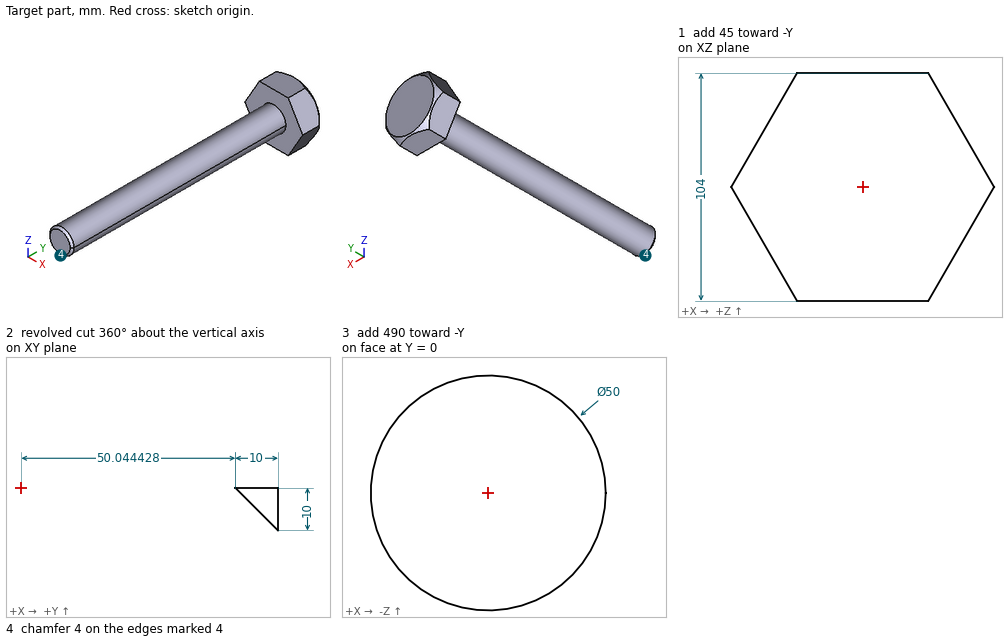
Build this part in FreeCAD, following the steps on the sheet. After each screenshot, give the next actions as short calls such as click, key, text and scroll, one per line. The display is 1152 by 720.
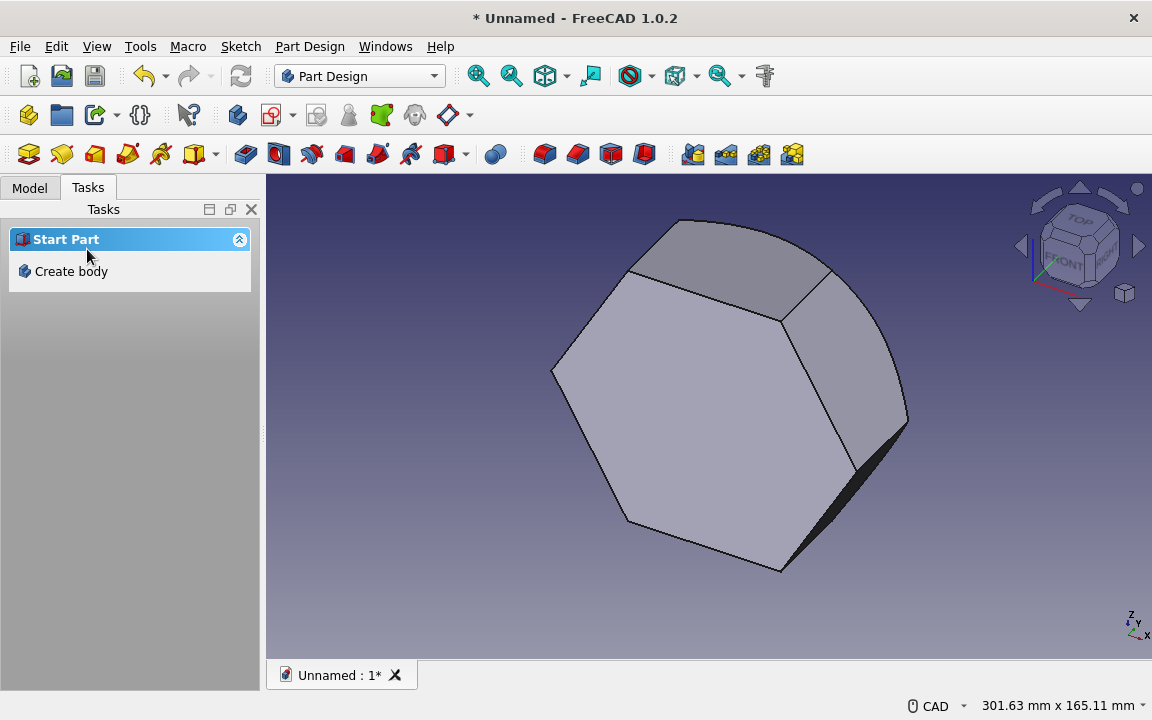
key(4)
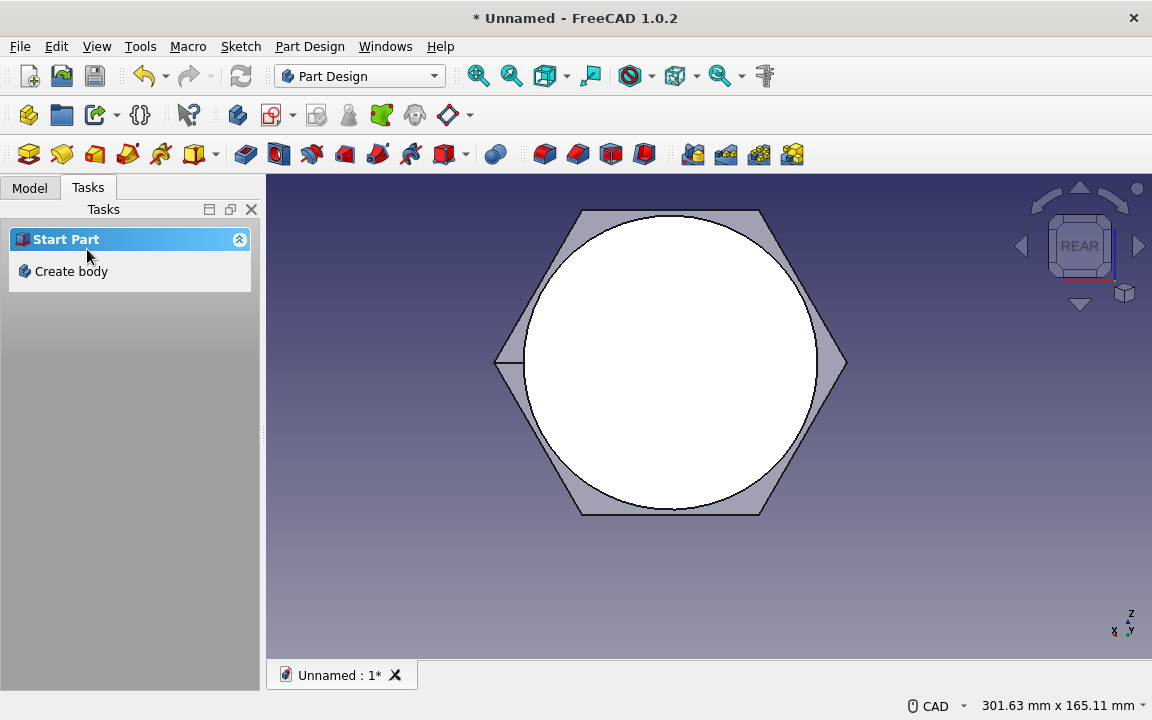
click(671, 362)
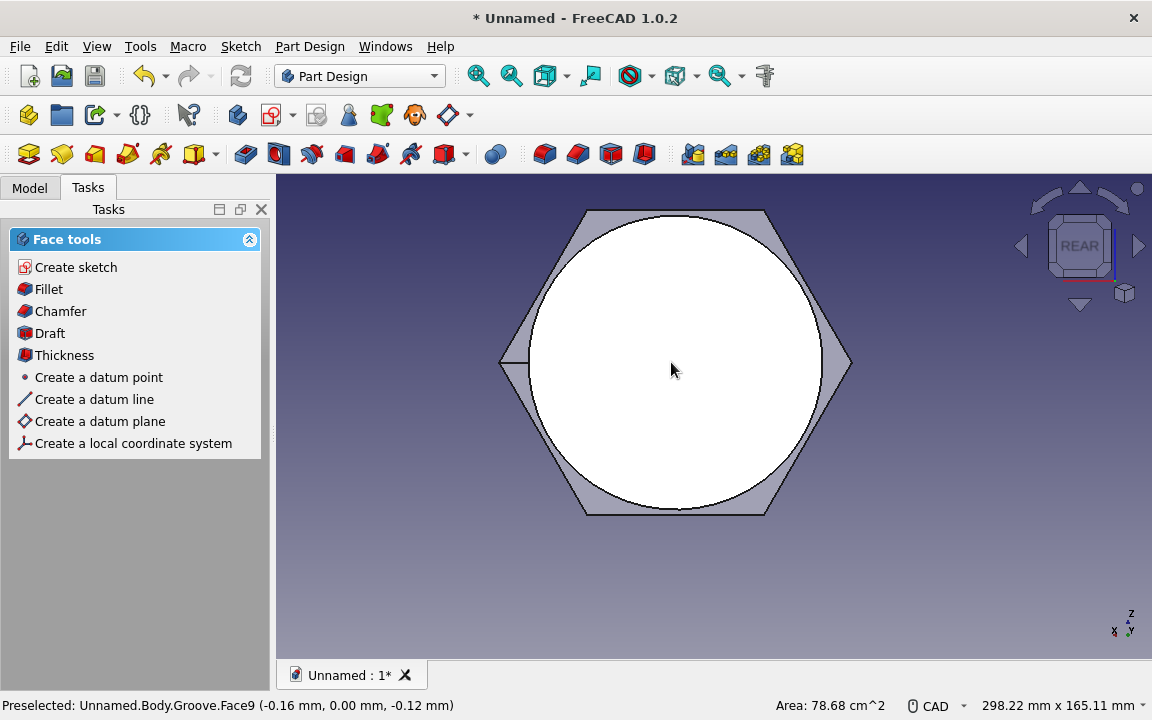
click(270, 116)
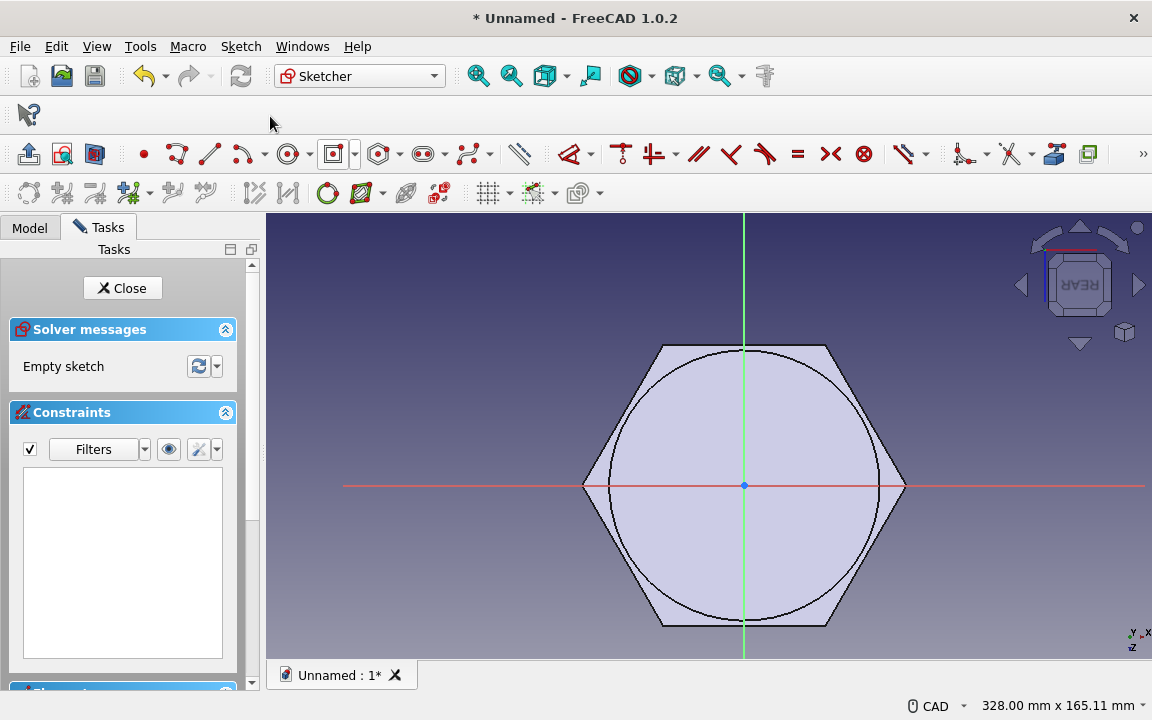
scroll(829, 526, up, 4)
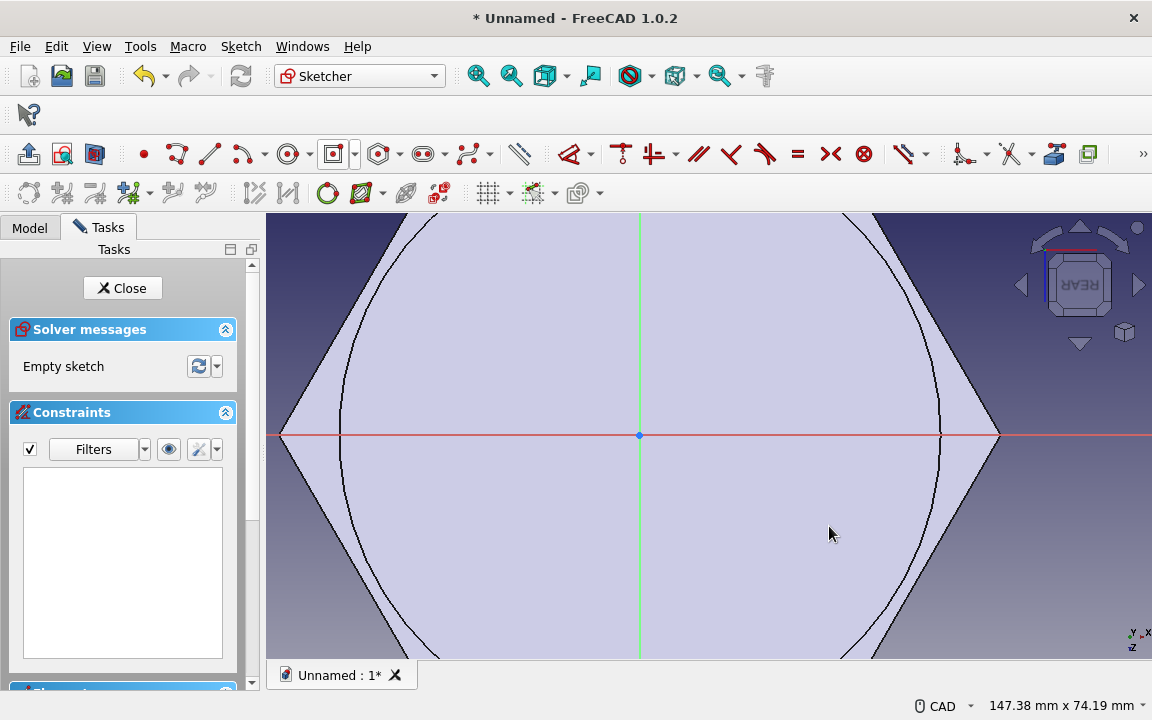
click(288, 154)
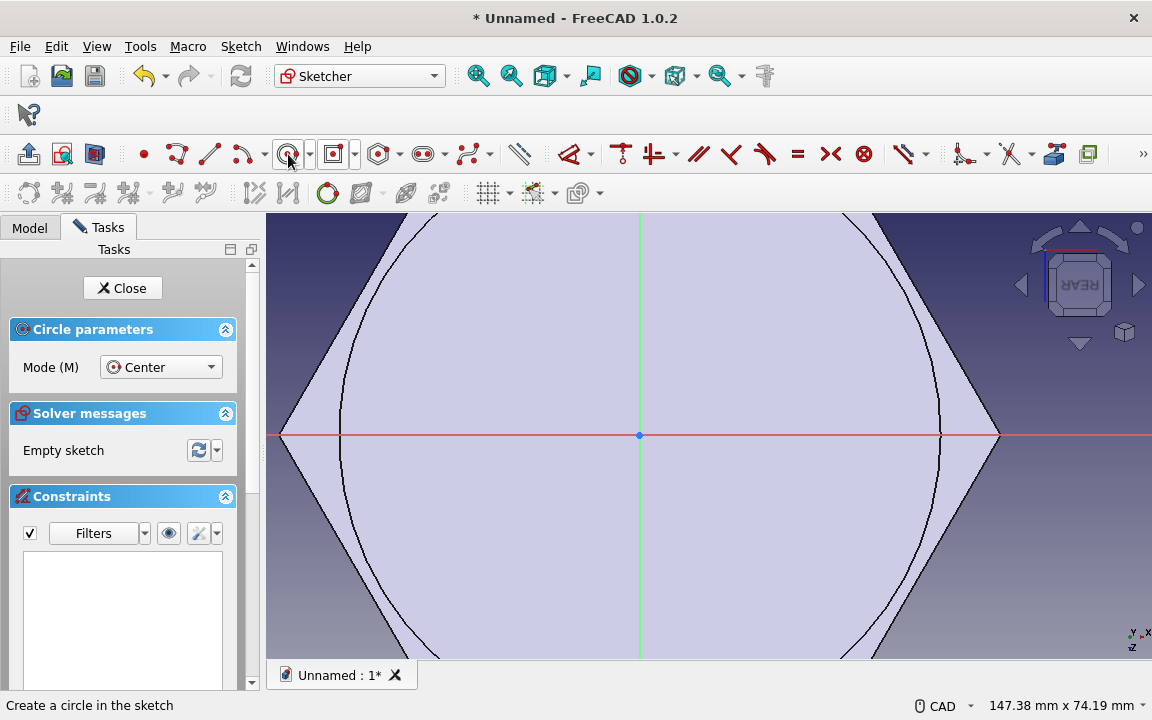
click(640, 435)
move(746, 329)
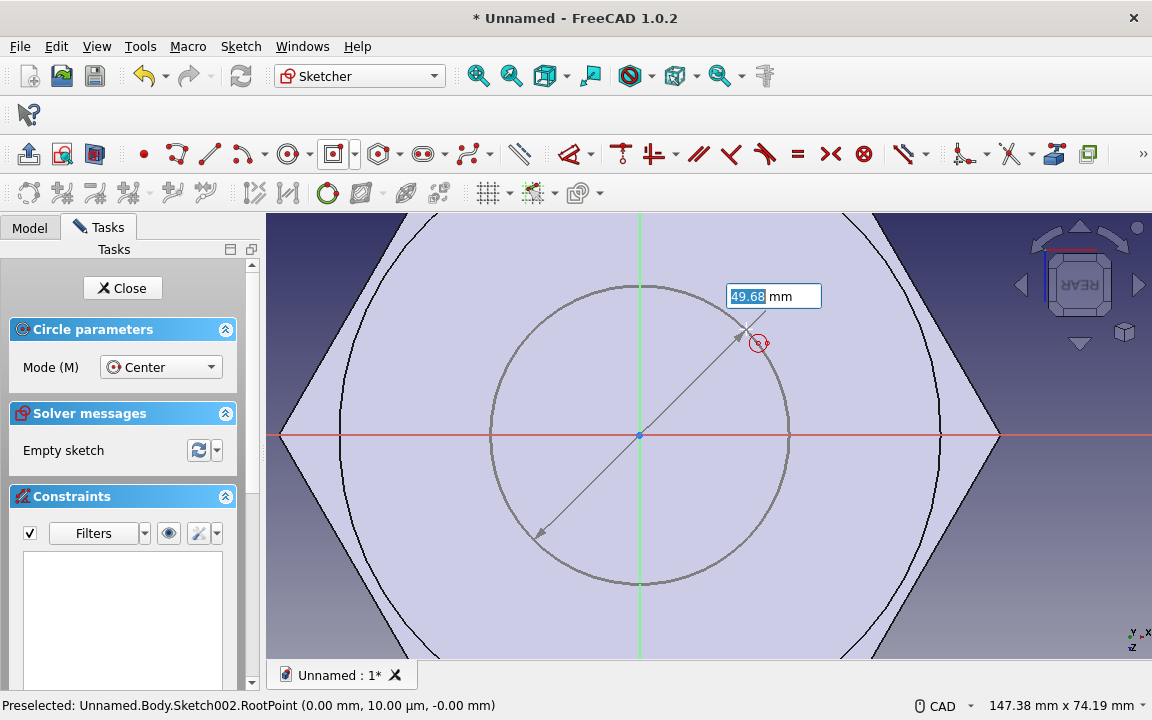
text(50)
key(Return)
key(Escape)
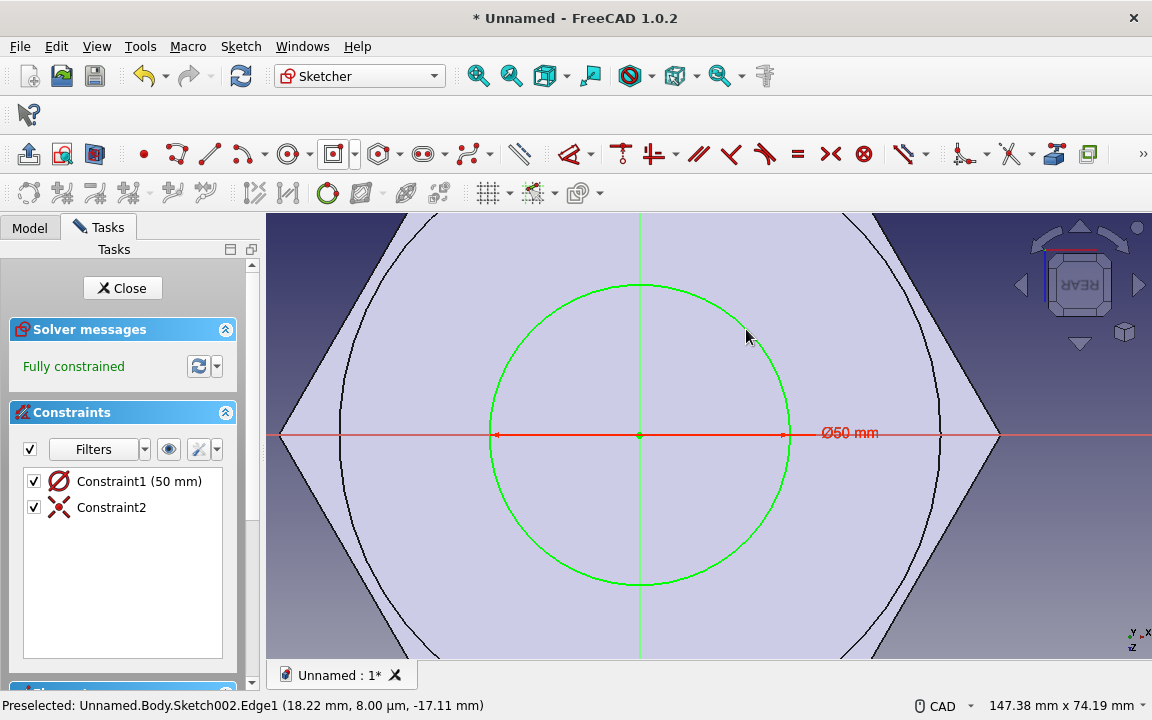
click(123, 288)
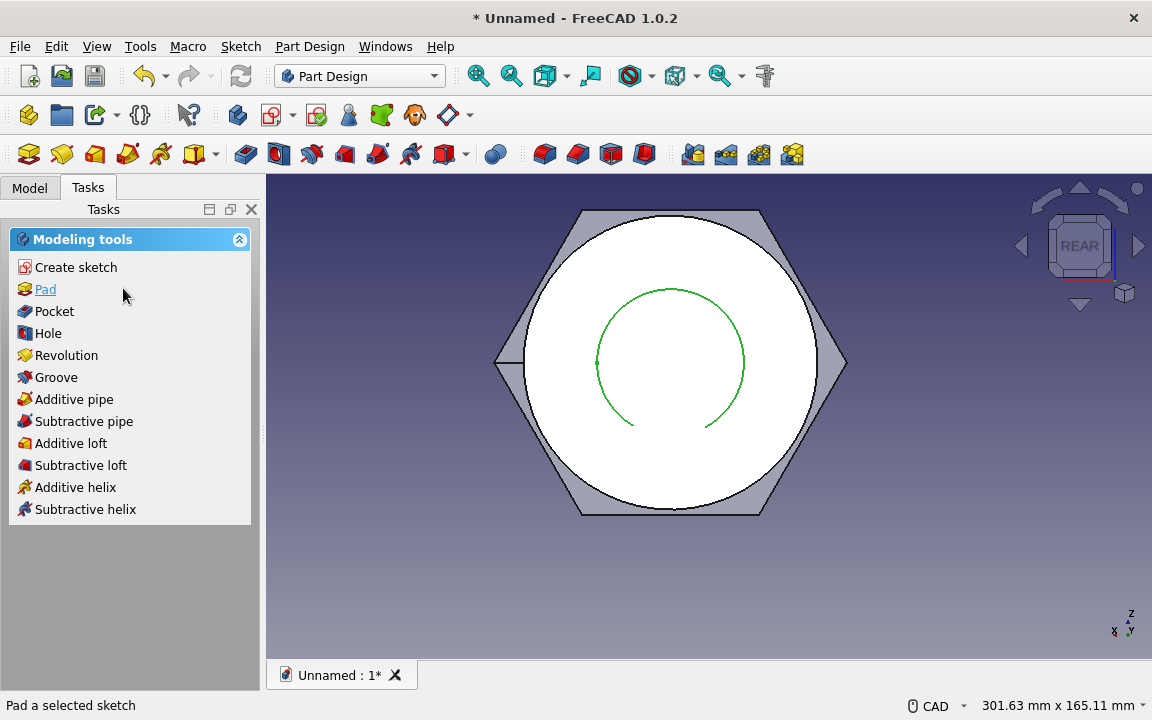
click(29, 154)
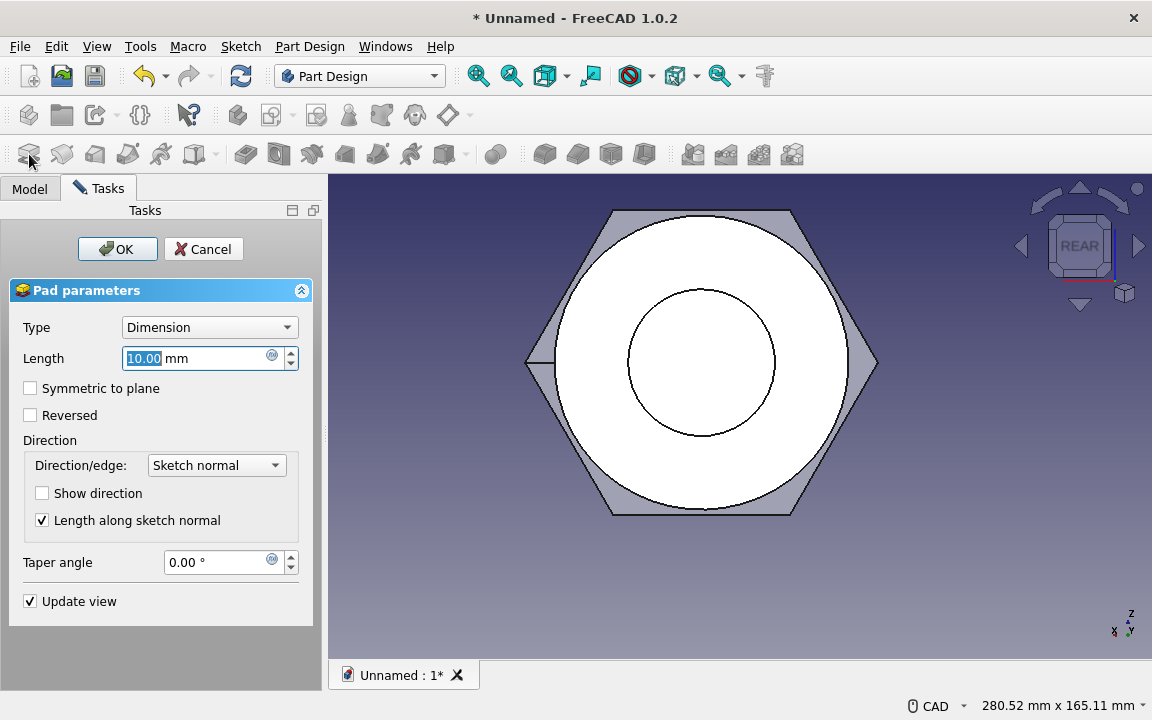
text(490)
key(Tab)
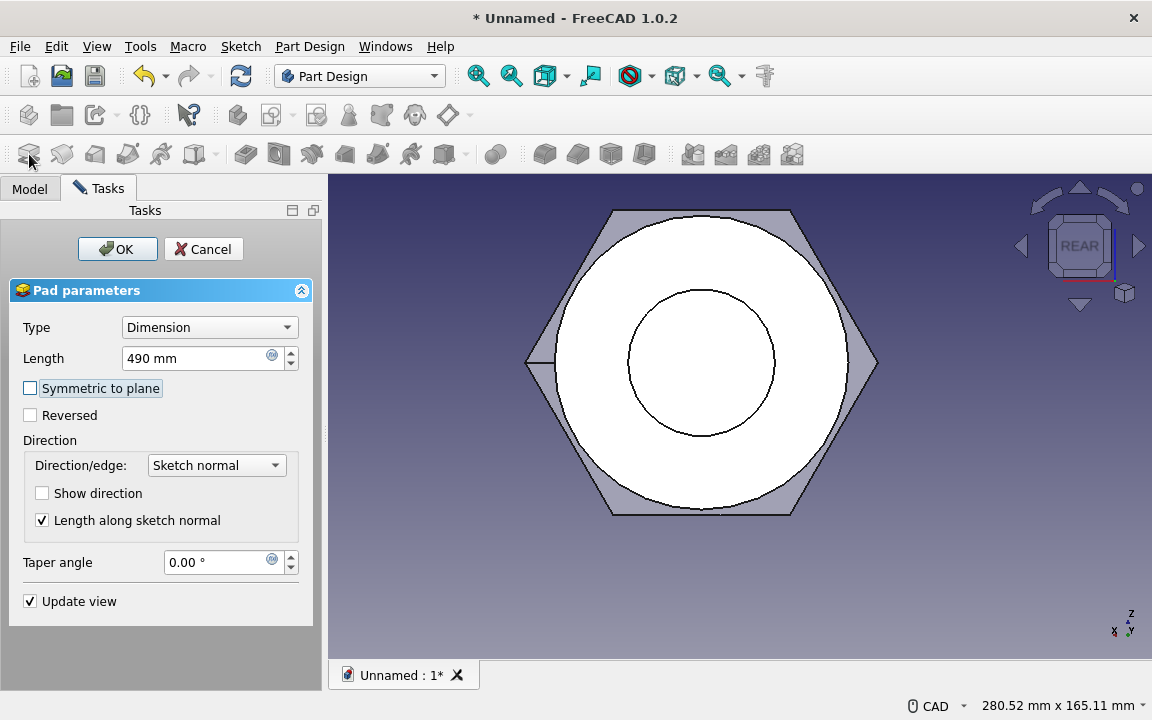
click(31, 415)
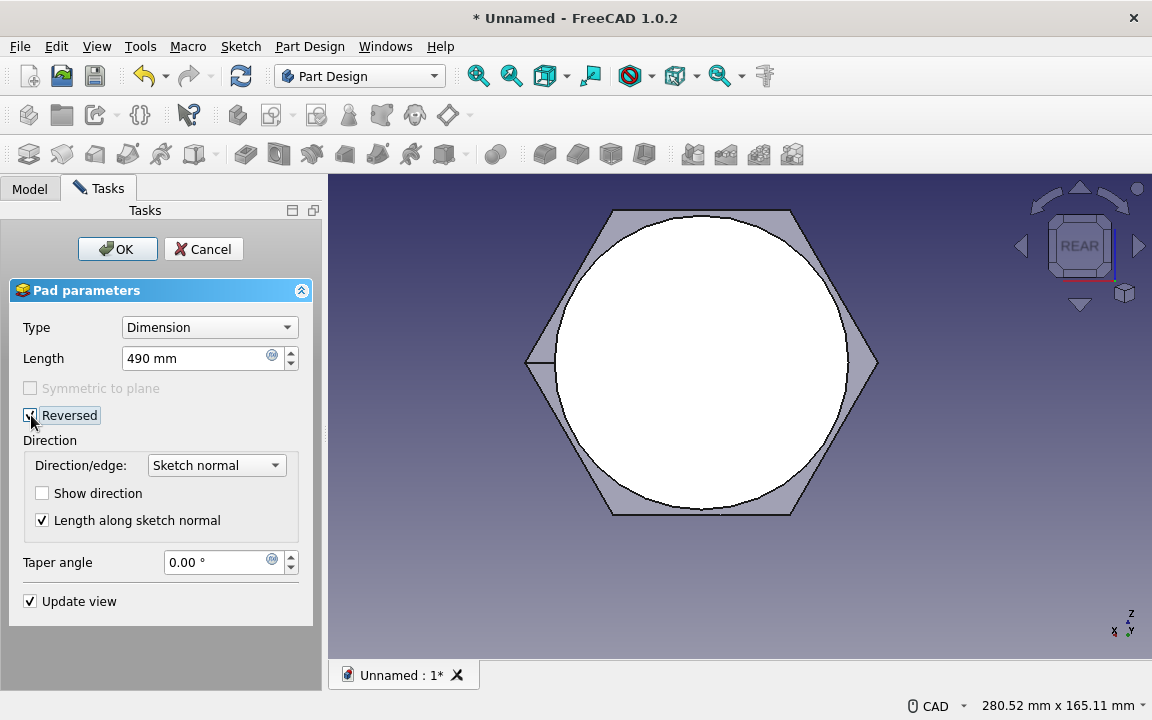
click(118, 249)